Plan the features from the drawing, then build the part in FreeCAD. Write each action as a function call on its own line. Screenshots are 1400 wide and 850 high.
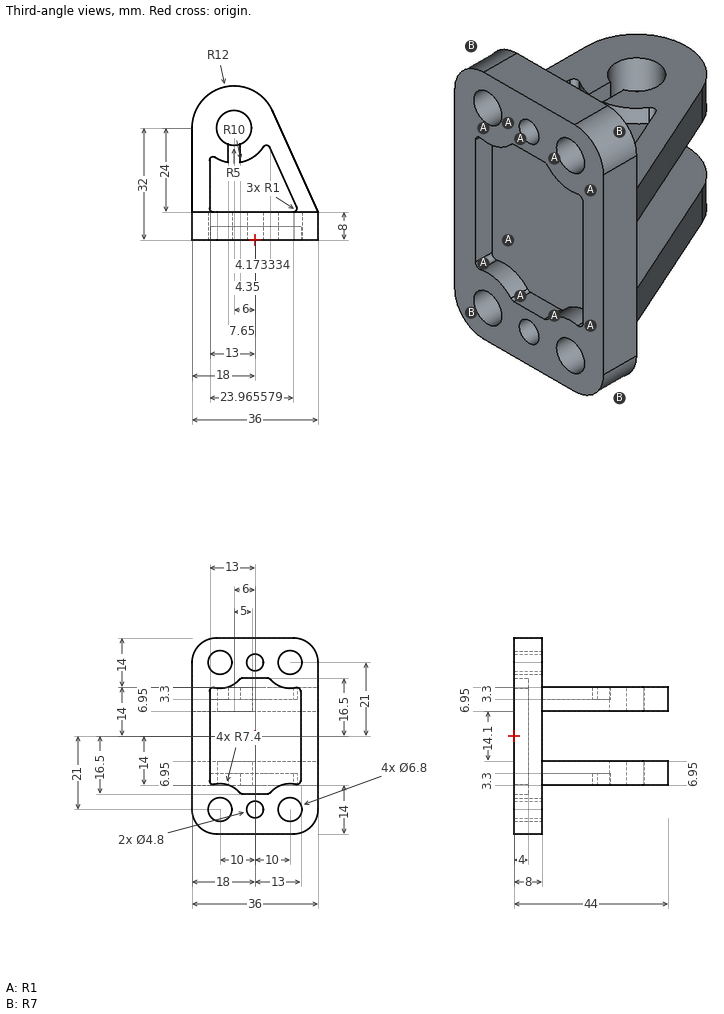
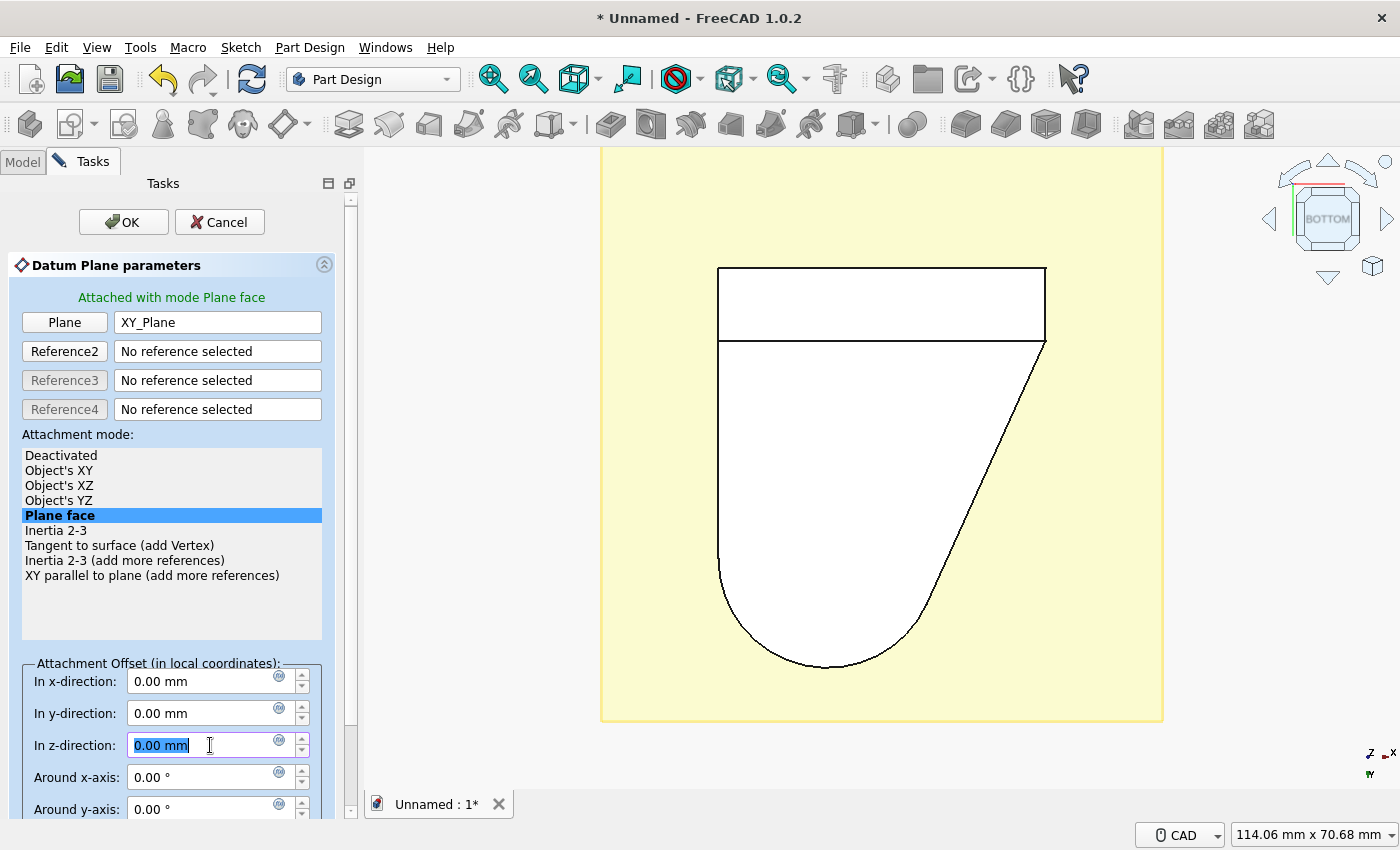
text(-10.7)
key(Tab)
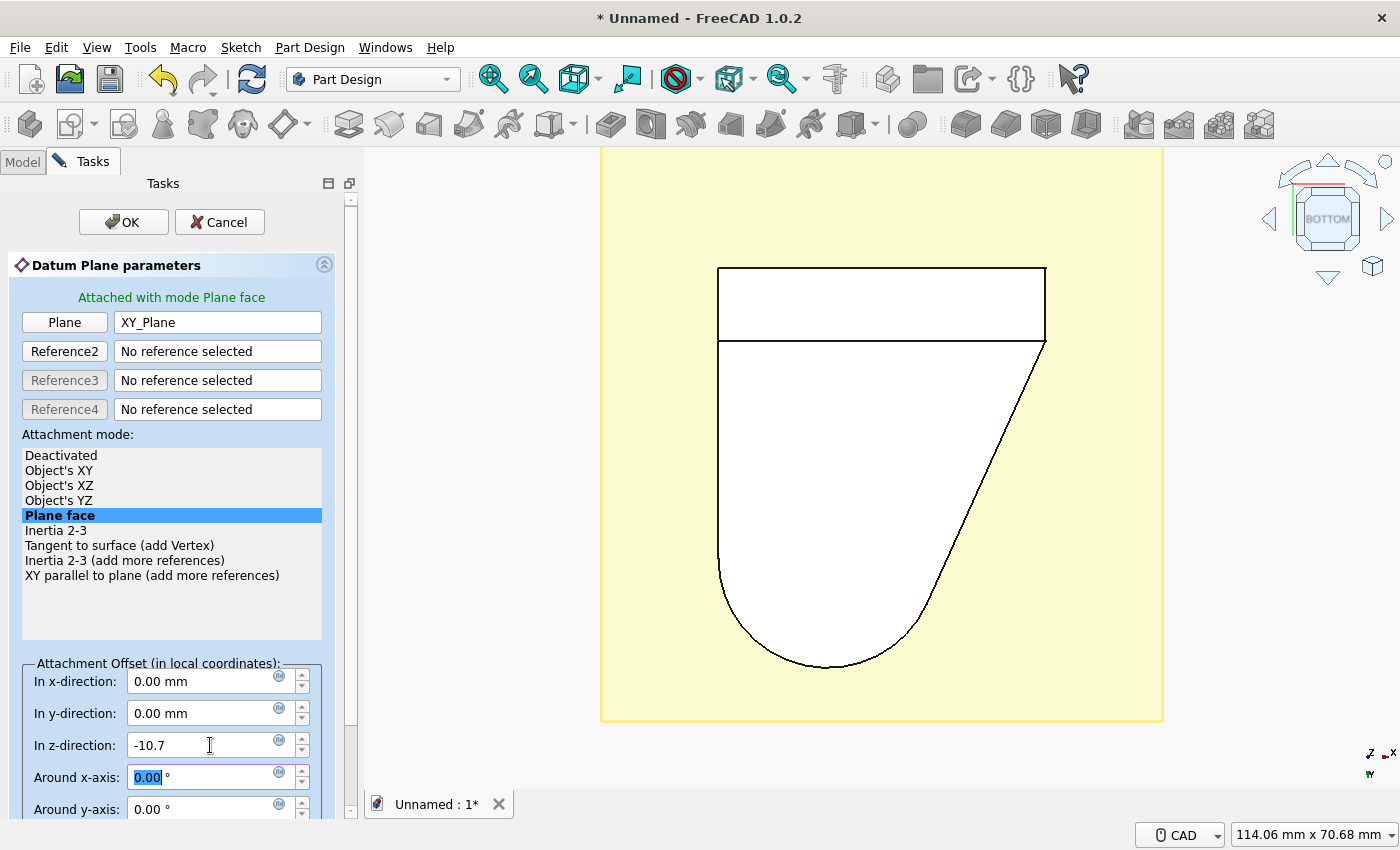
click(124, 222)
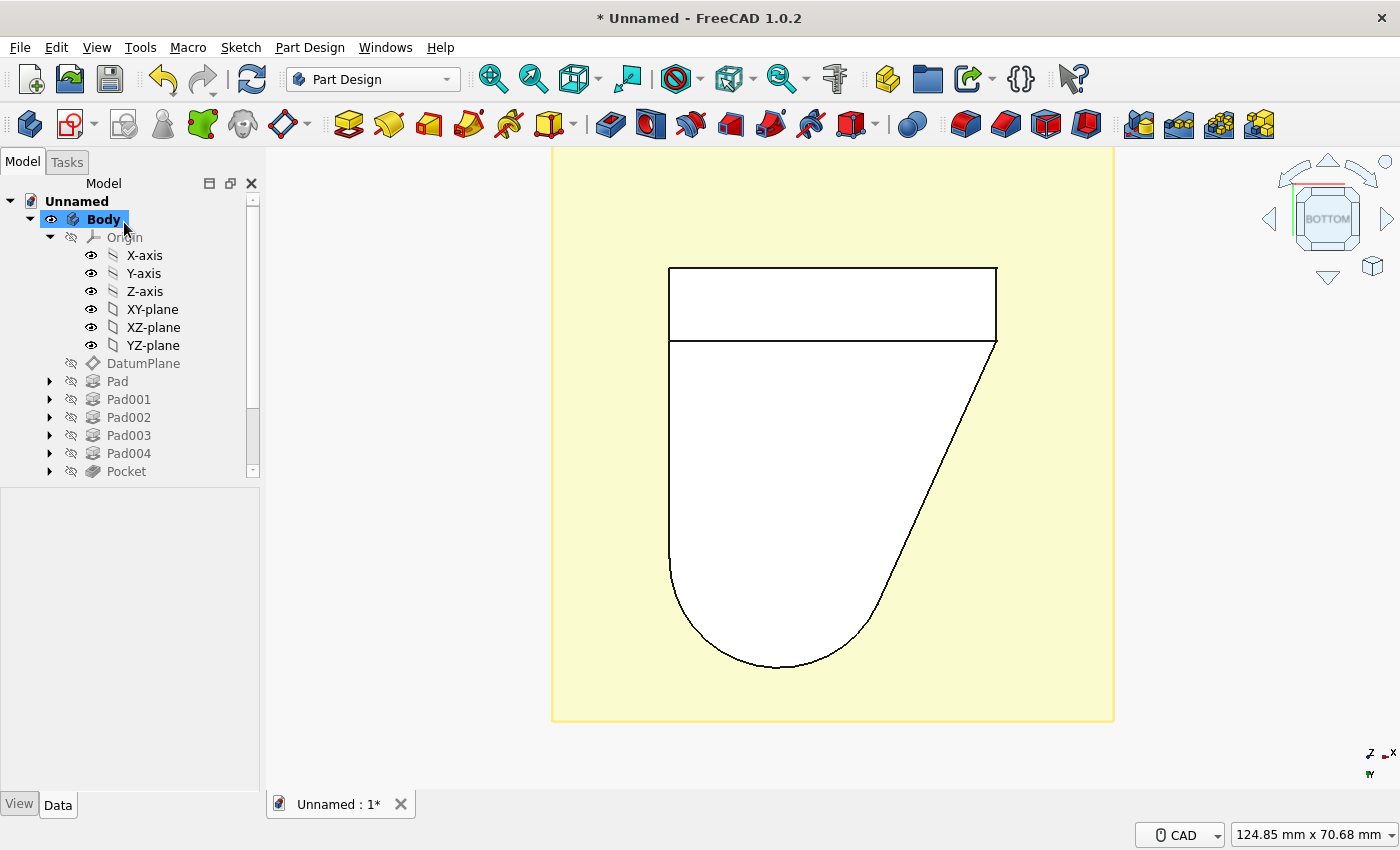
scroll(100, 341, down, 3)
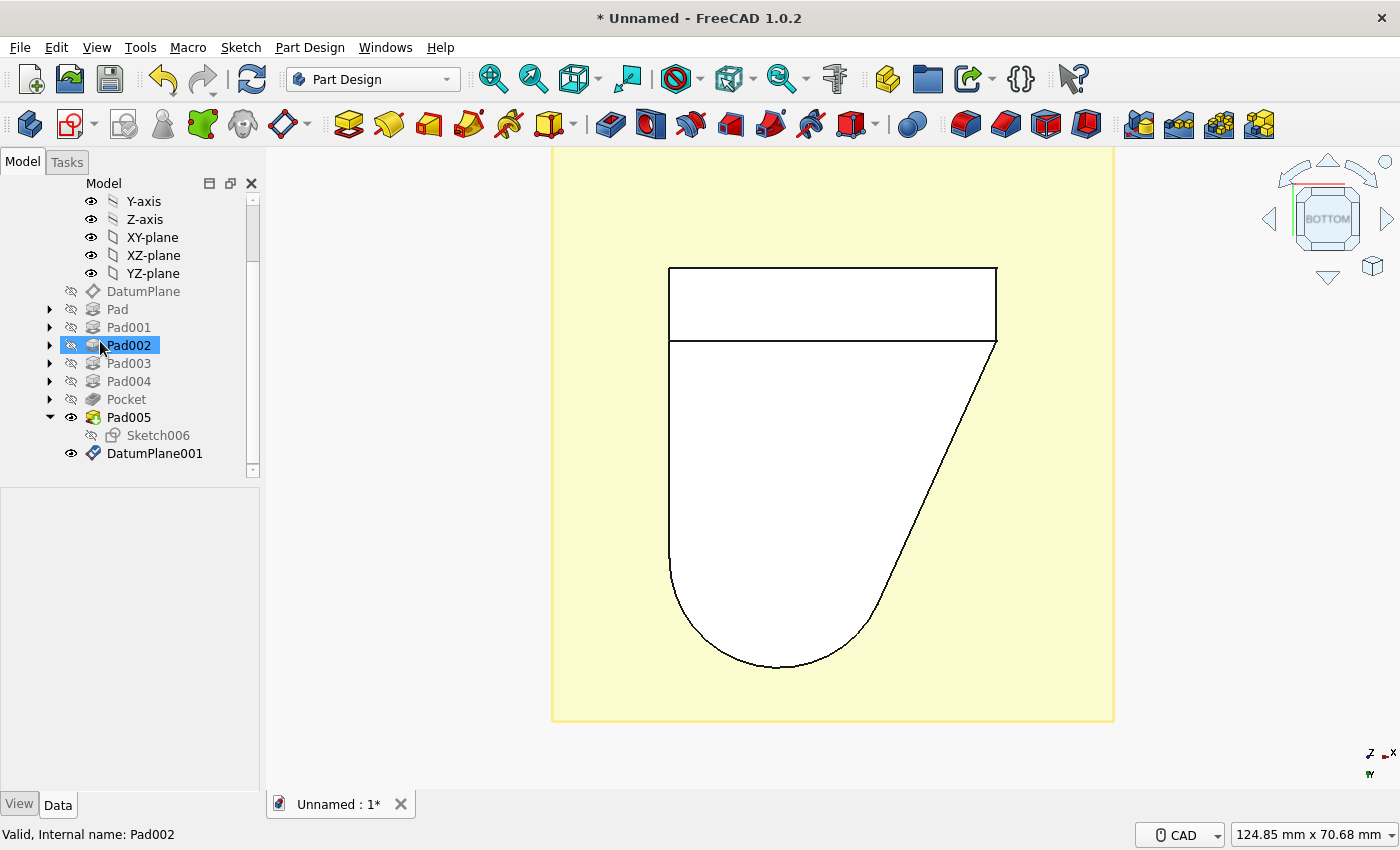
click(116, 453)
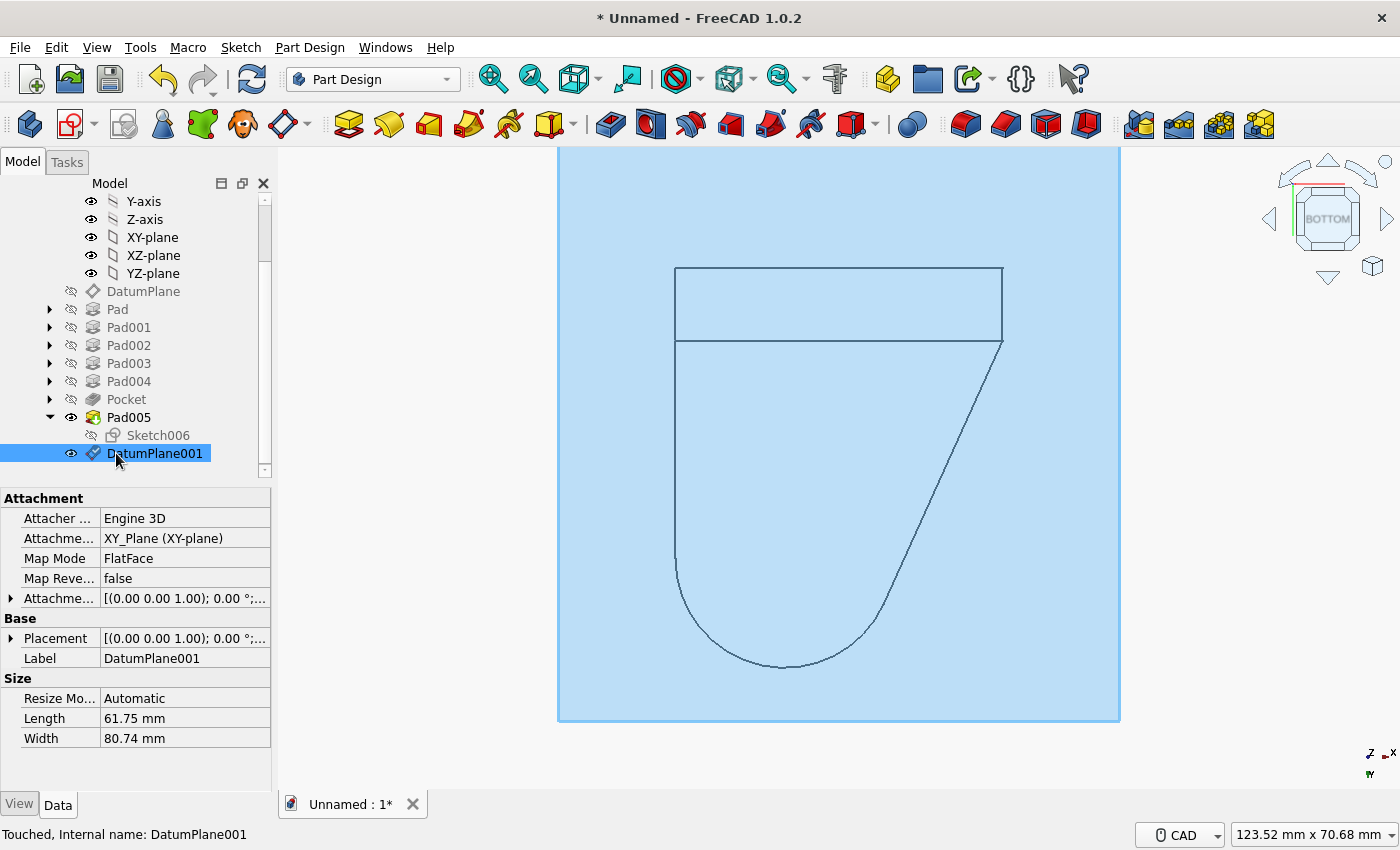
click(70, 124)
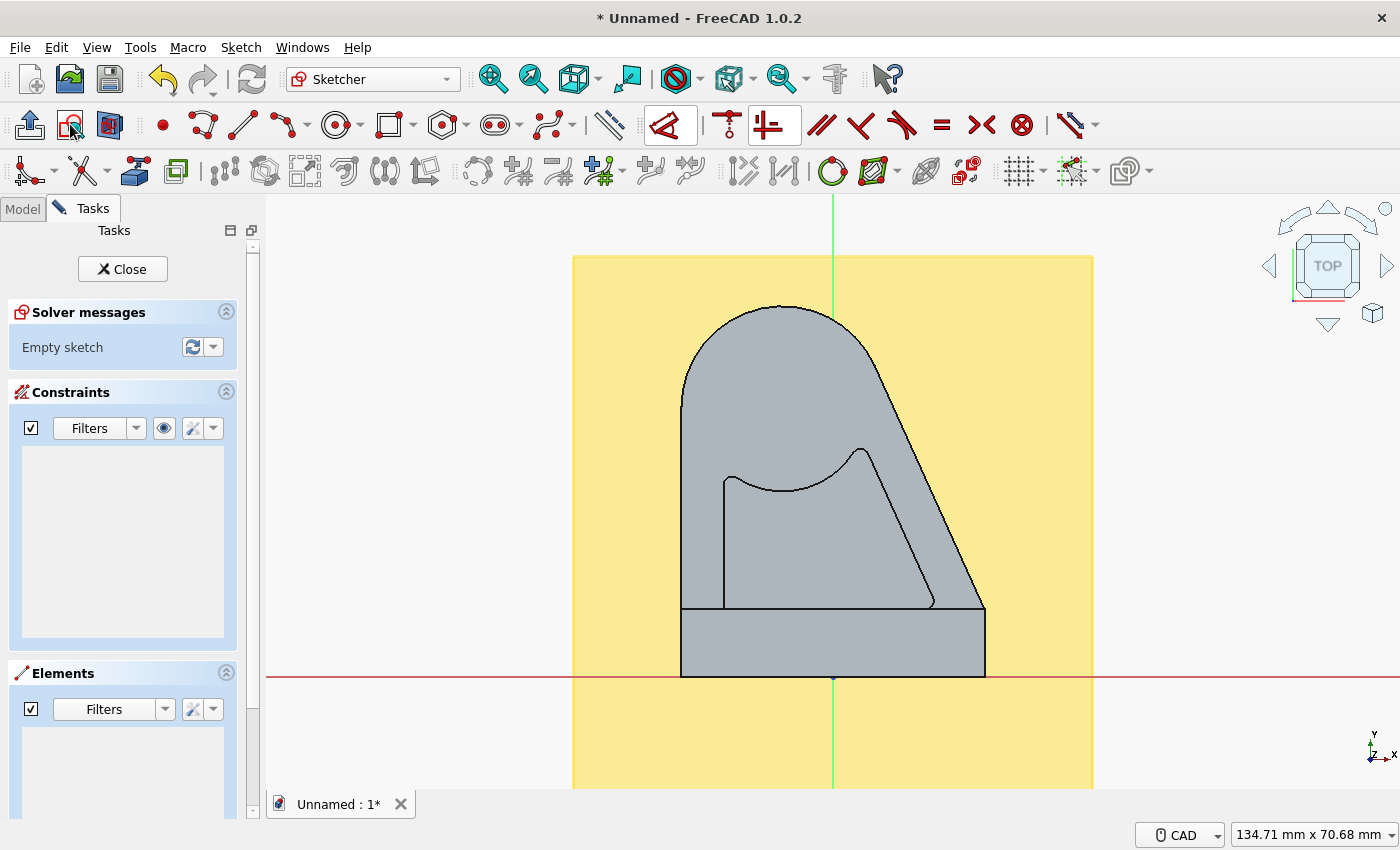
click(110, 126)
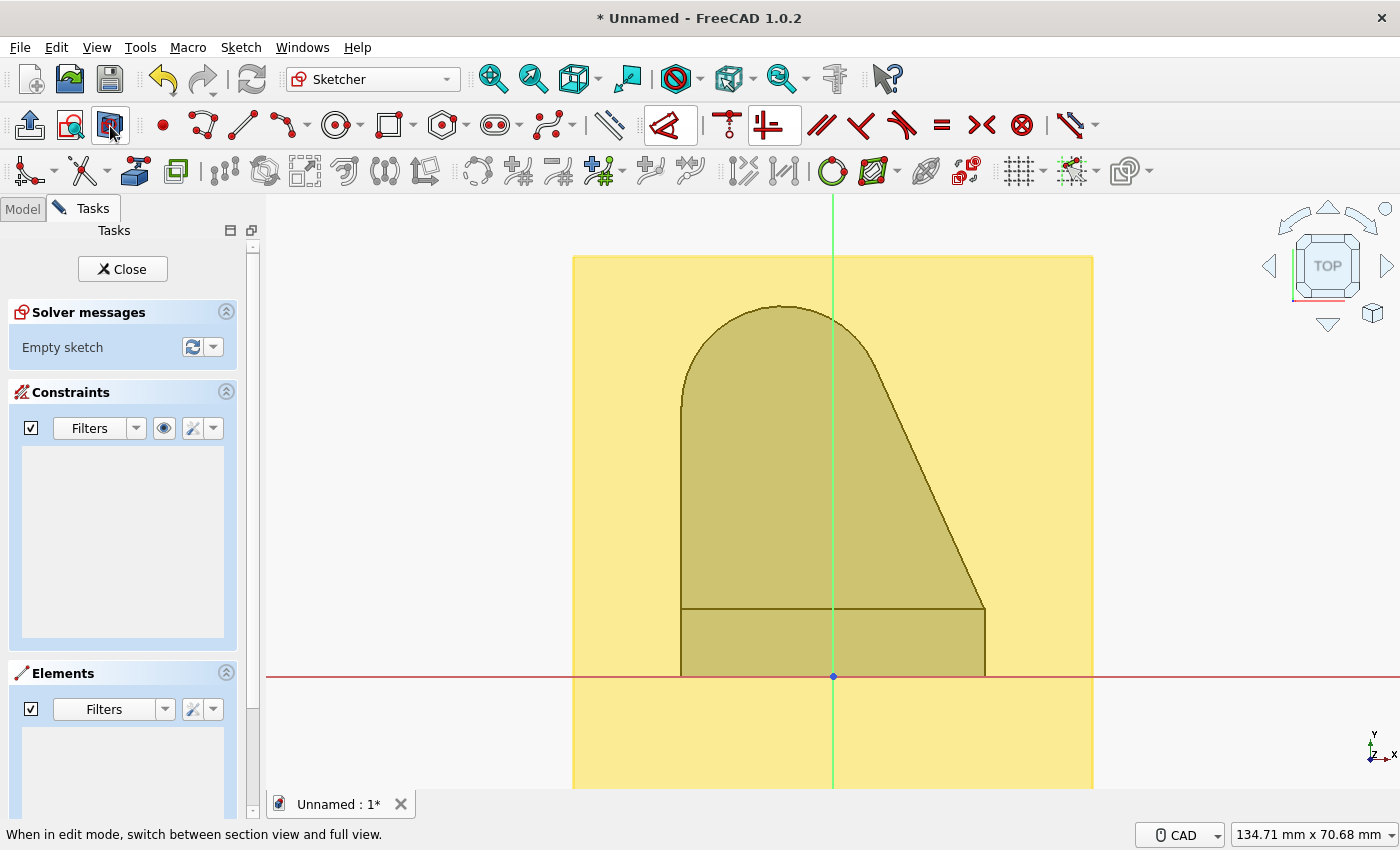
scroll(906, 649, up, 3)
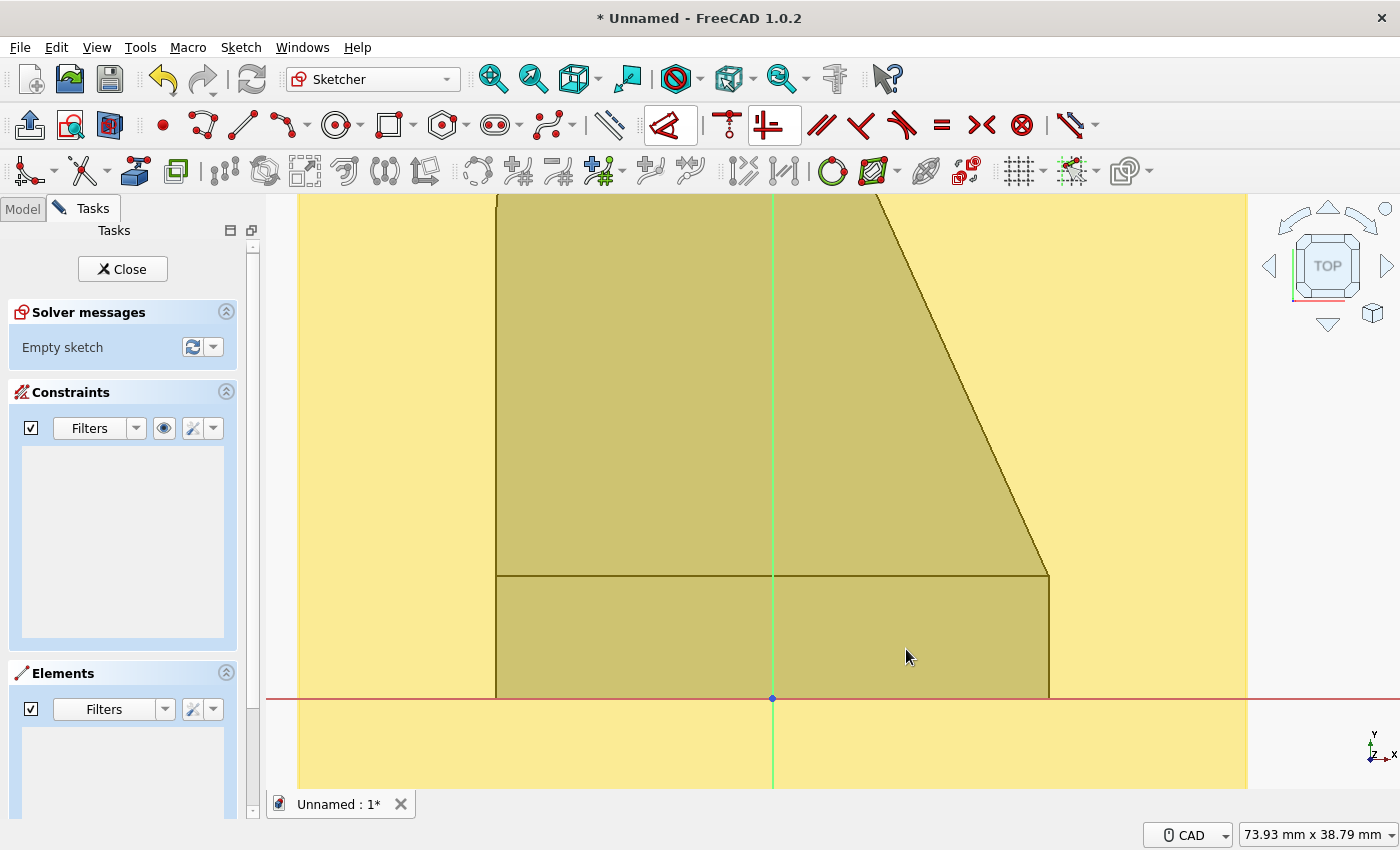
click(244, 126)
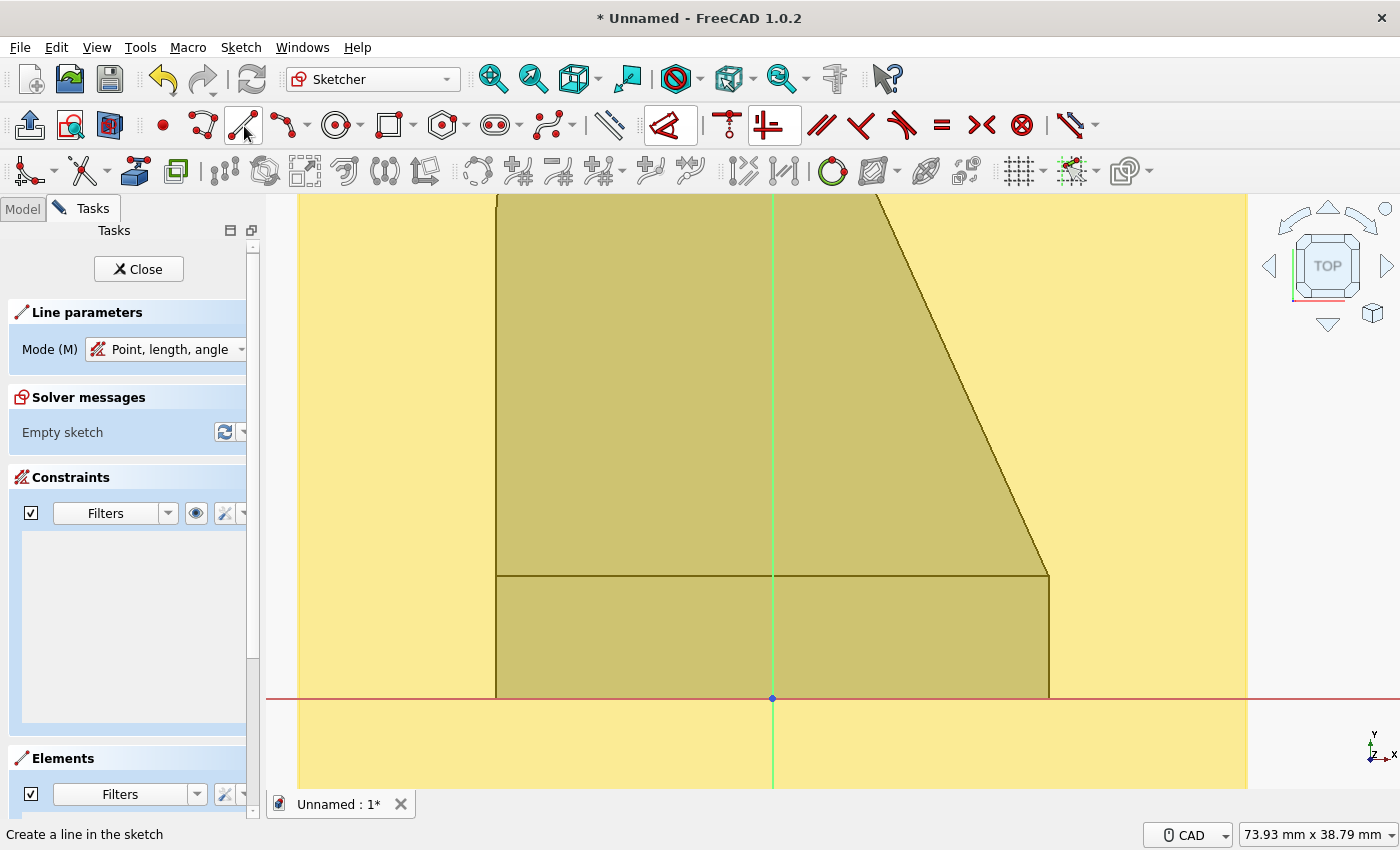
click(837, 293)
click(955, 554)